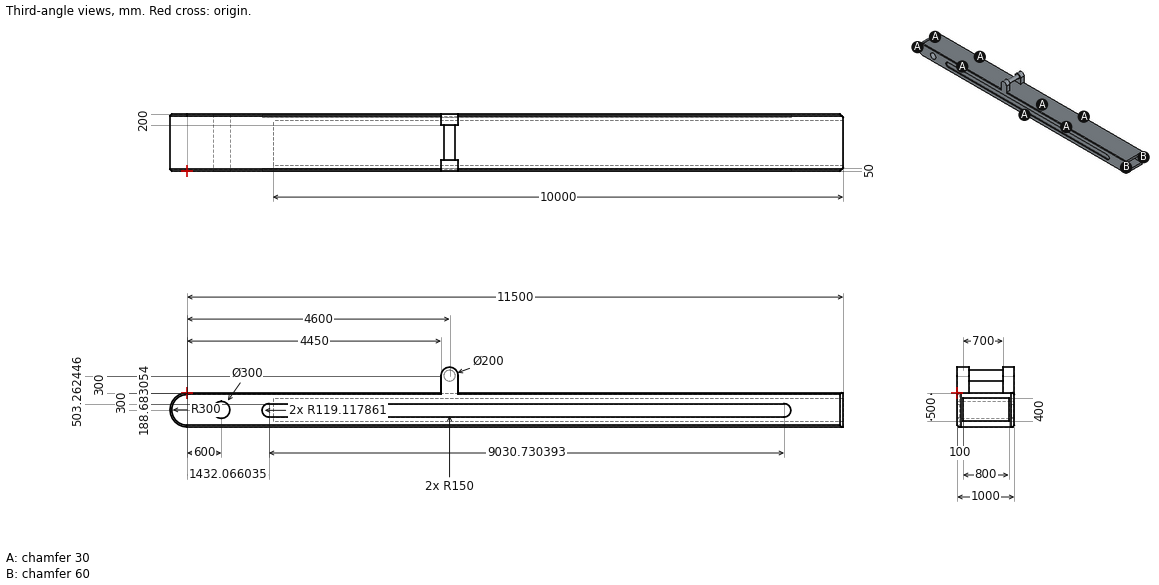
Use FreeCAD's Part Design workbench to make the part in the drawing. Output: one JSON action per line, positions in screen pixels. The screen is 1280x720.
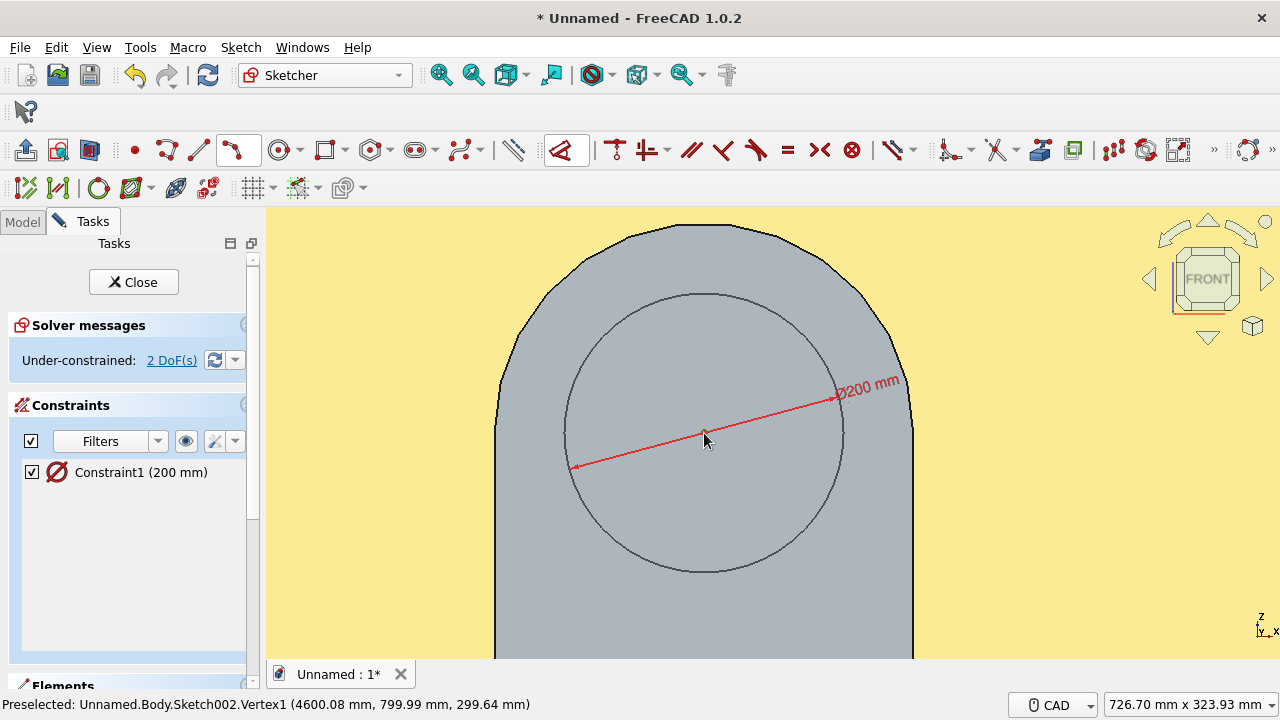
{"action": "key", "text": "i"}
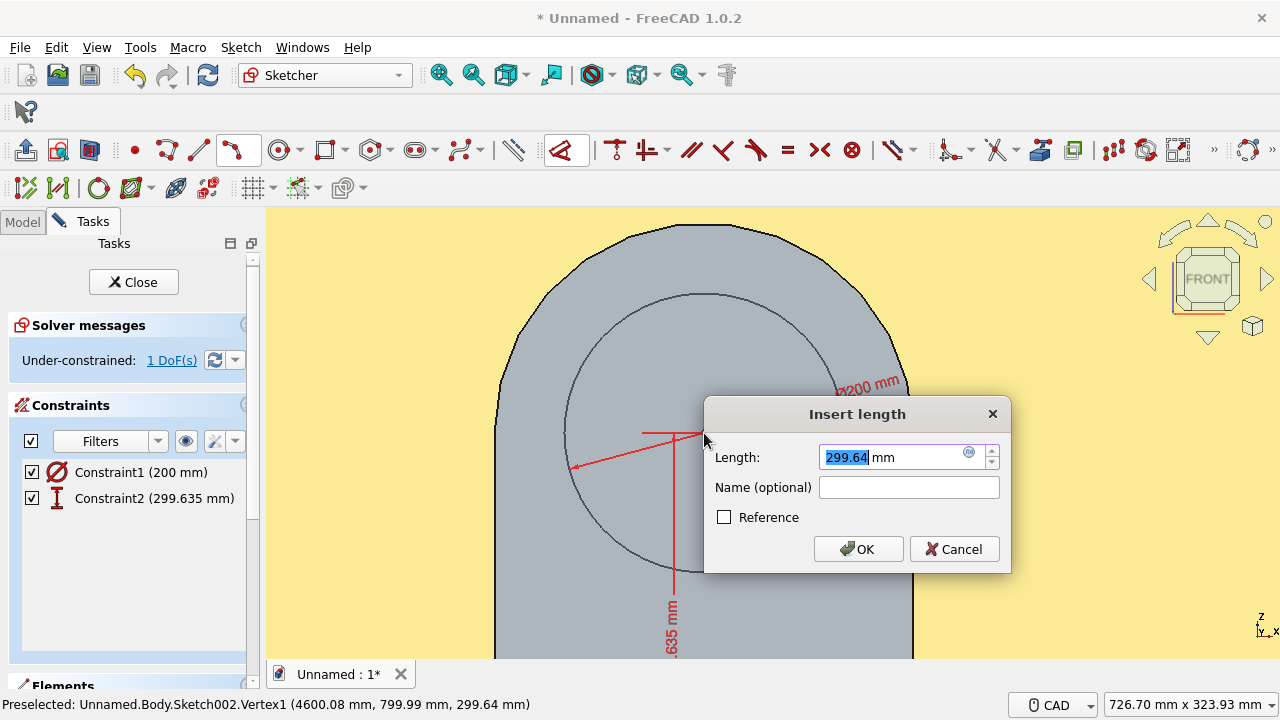
{"action": "type", "text": "300"}
{"action": "key", "text": "Return"}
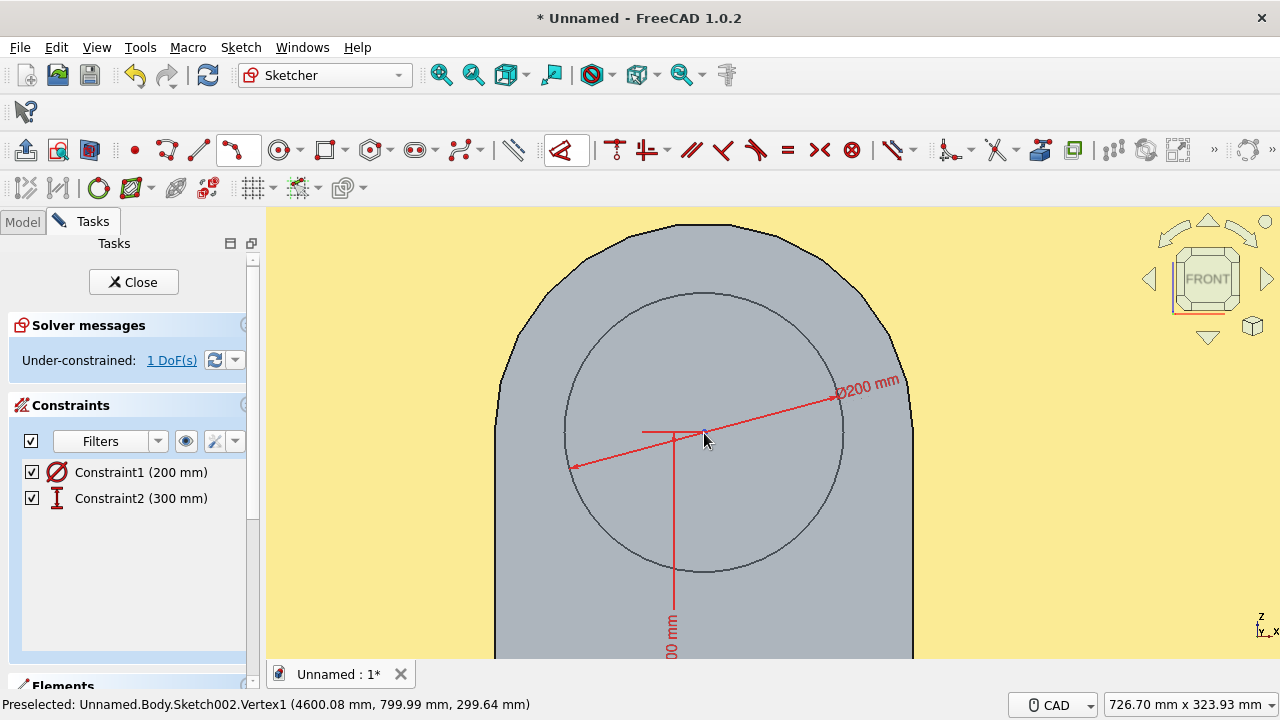
{"action": "left_click", "coordinate": [704, 432]}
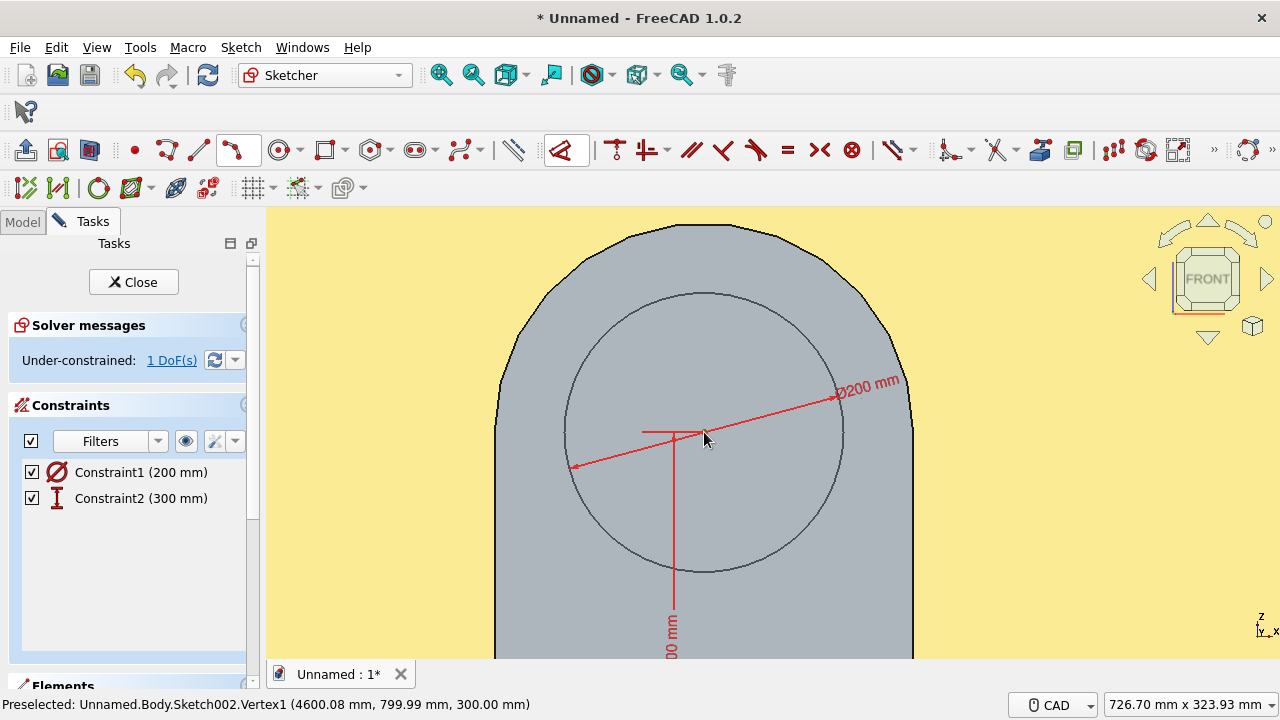
{"action": "key", "text": "l"}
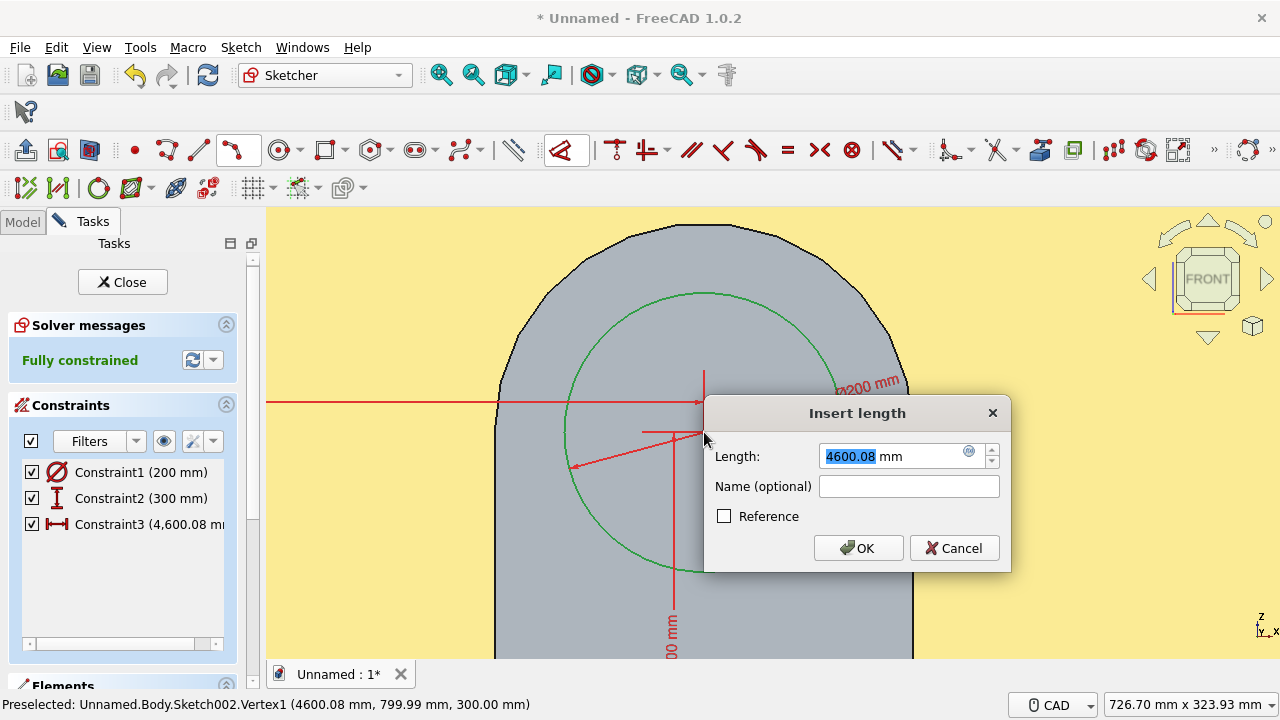
{"action": "type", "text": "4600"}
{"action": "key", "text": "Return"}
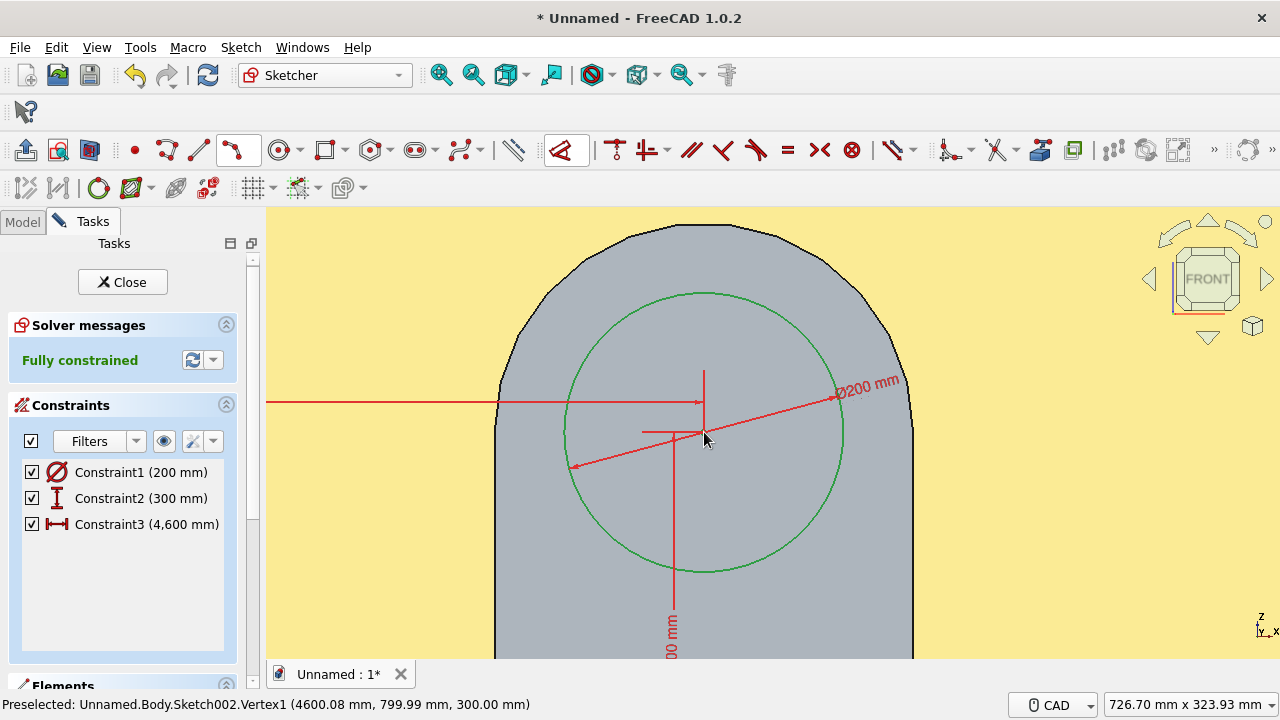
{"action": "left_click", "coordinate": [123, 282]}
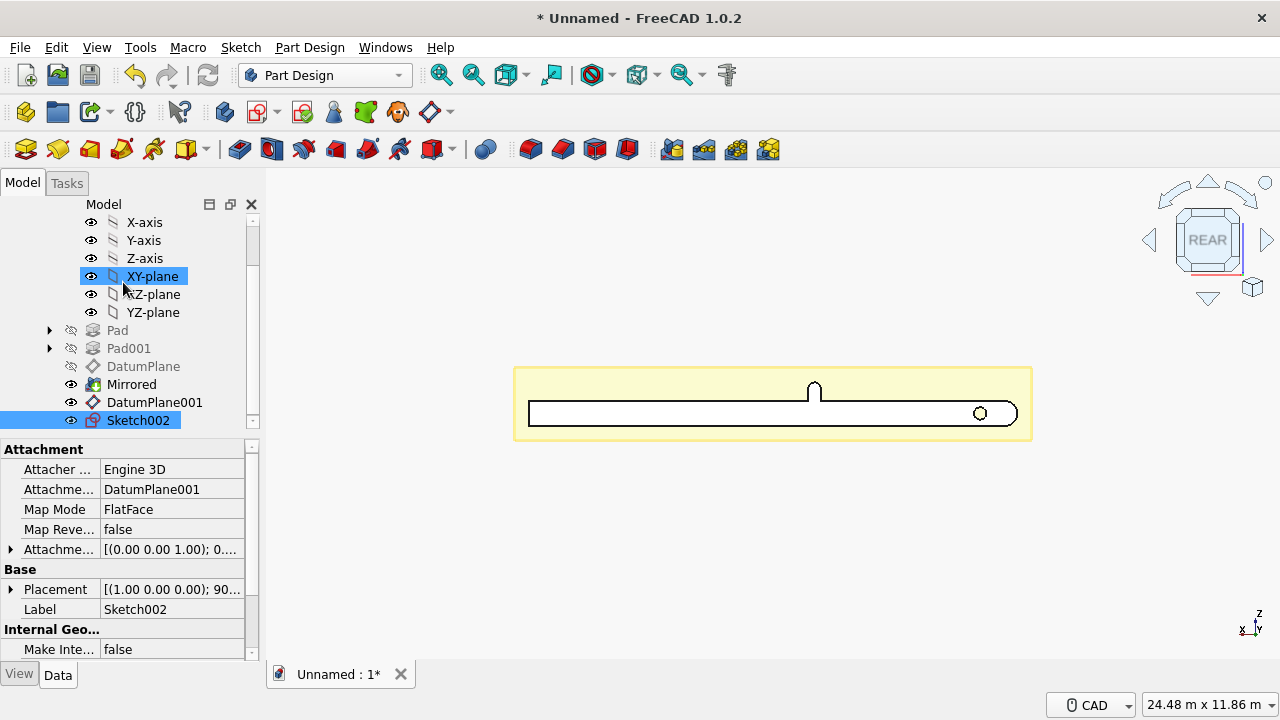
{"action": "left_click", "coordinate": [26, 150]}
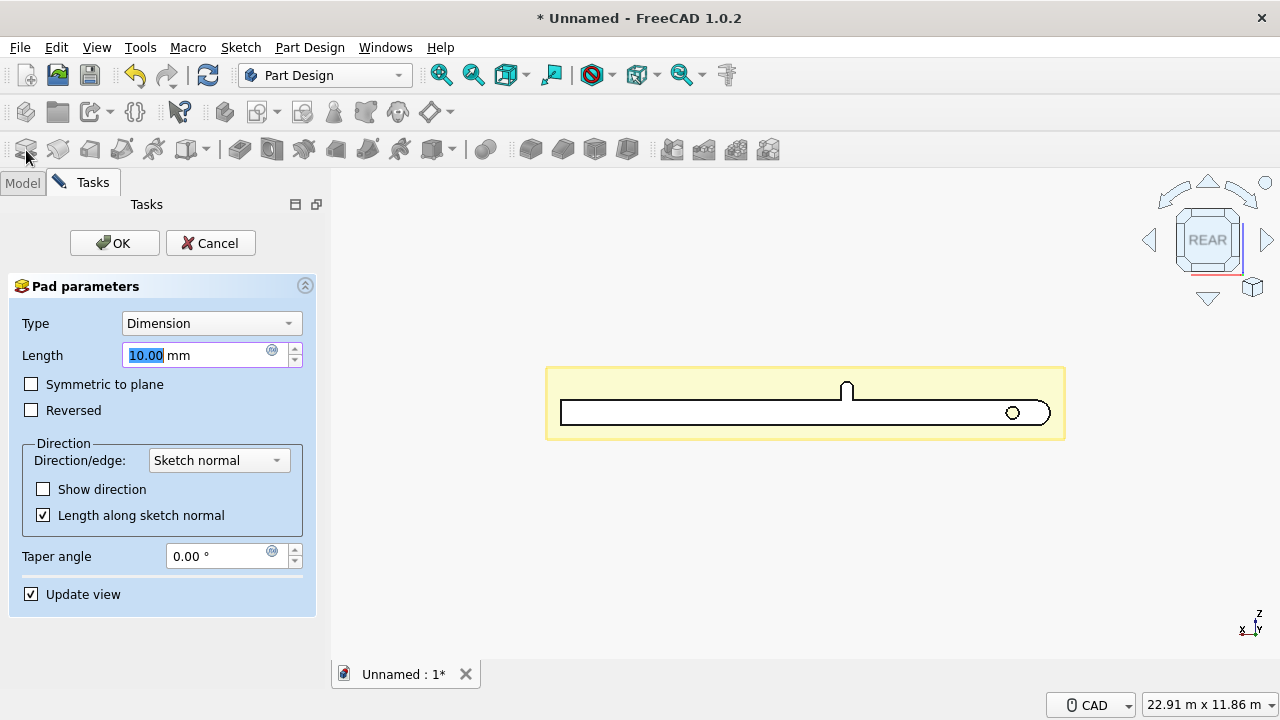
{"action": "type", "text": "700"}
{"action": "key", "text": "Tab"}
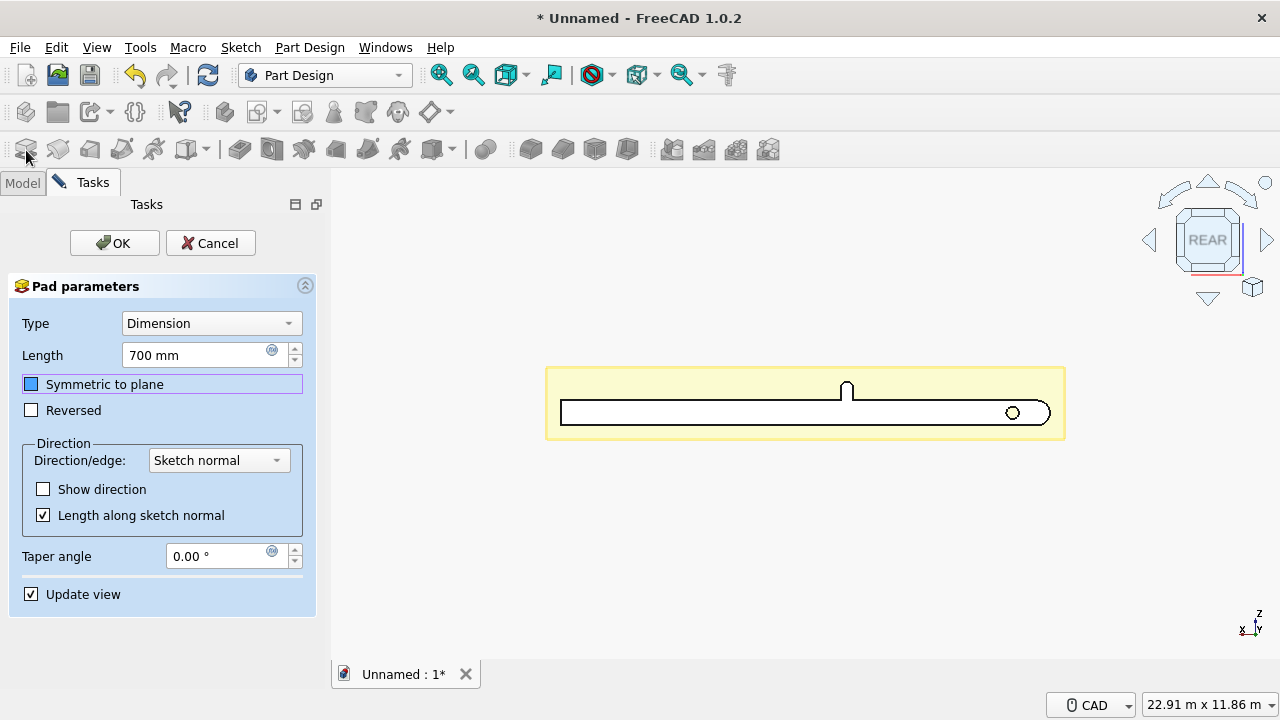
{"action": "left_click", "coordinate": [115, 243]}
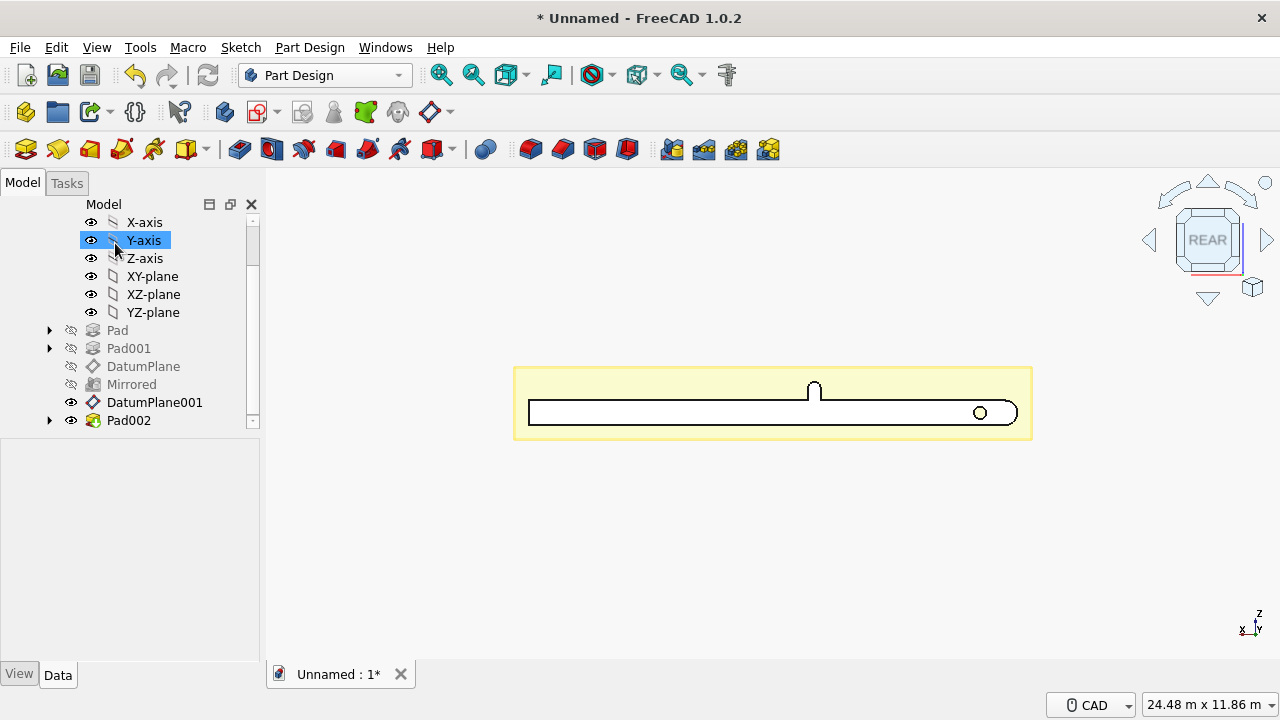
{"action": "left_click", "coordinate": [116, 402]}
{"action": "key", "text": "space"}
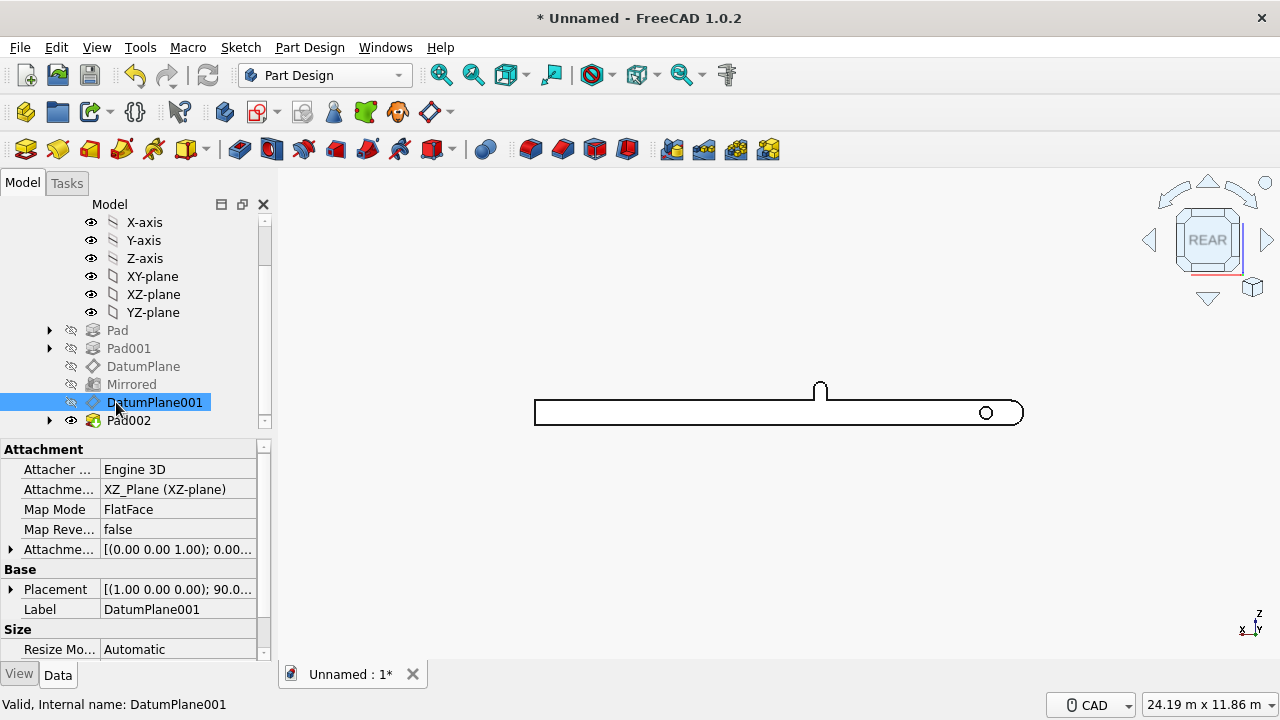
{"action": "key", "text": "0"}